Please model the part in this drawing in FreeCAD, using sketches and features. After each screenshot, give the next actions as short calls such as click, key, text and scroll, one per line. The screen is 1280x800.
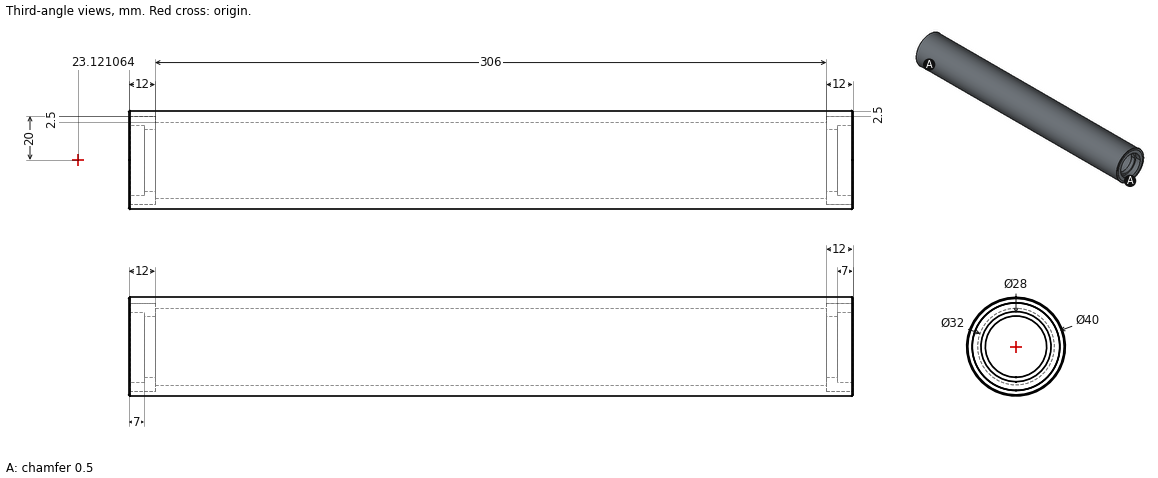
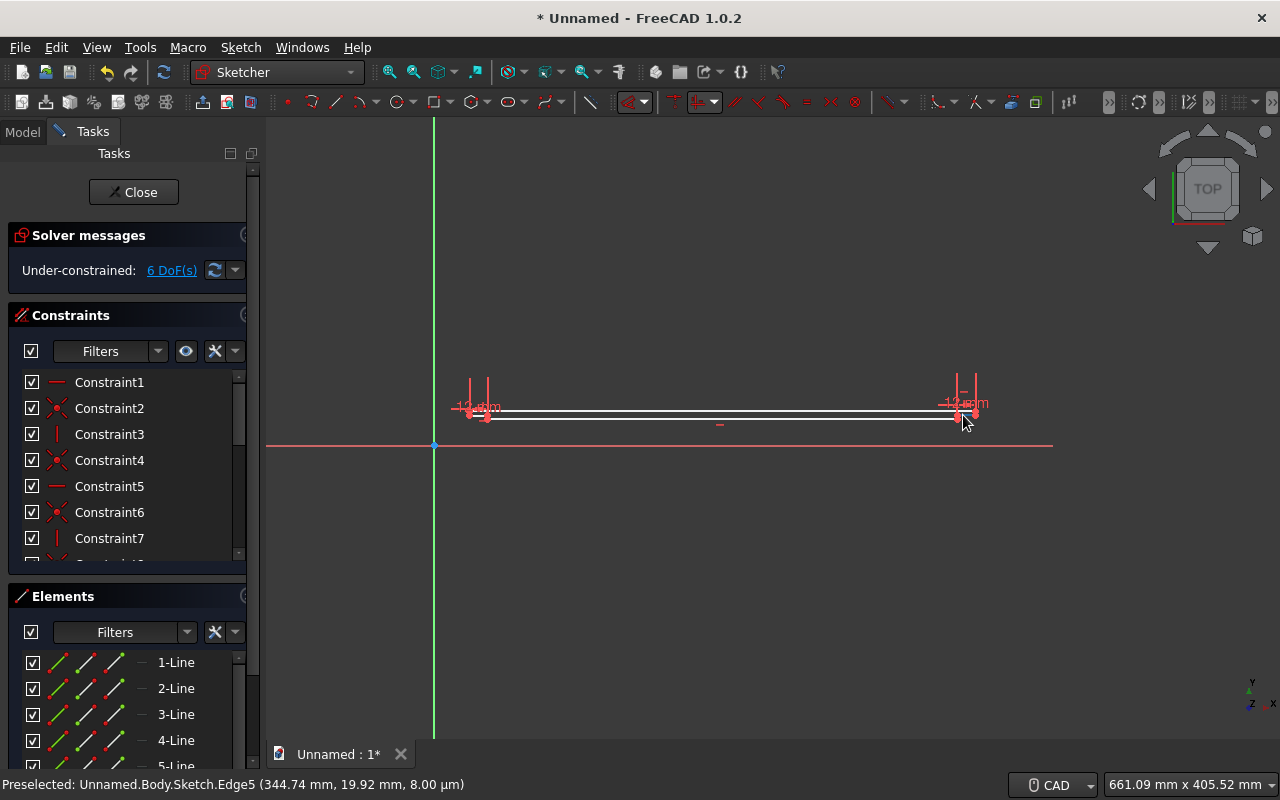
scroll(488, 418, up, 12)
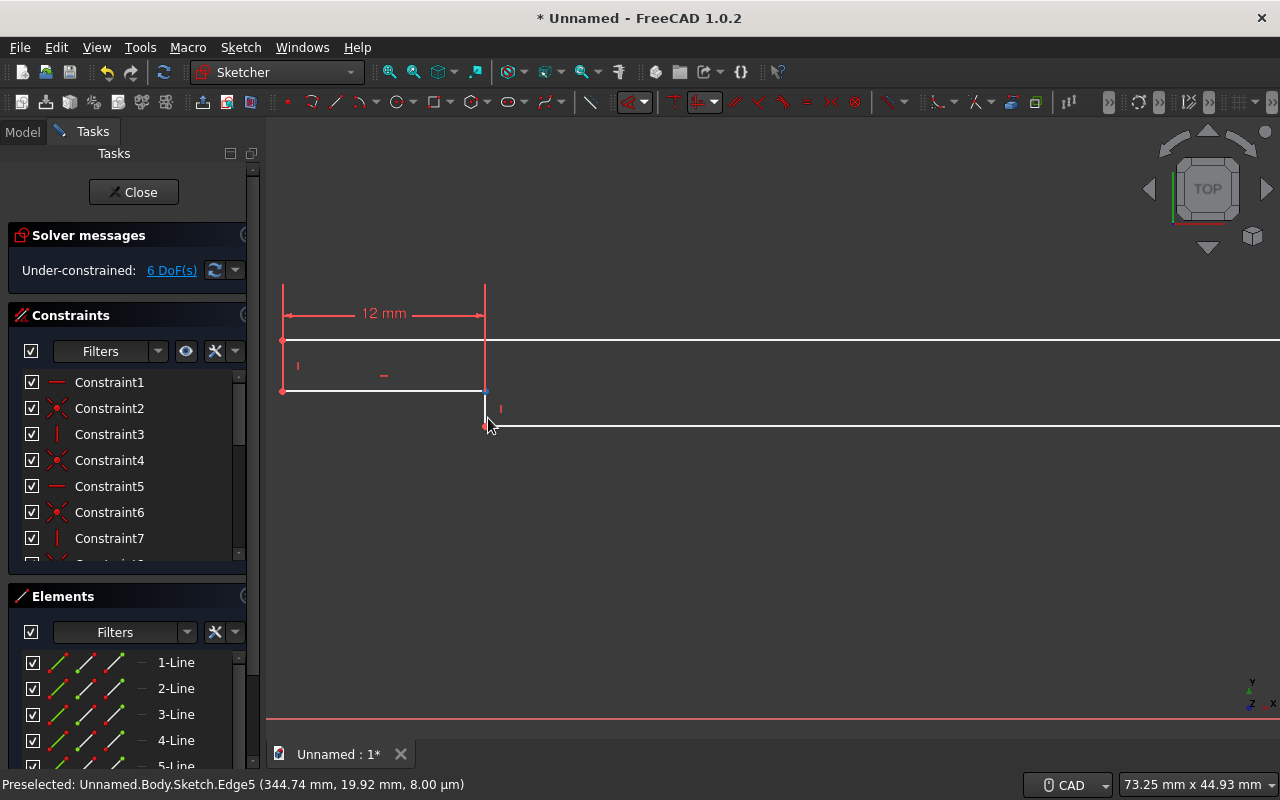
click(485, 409)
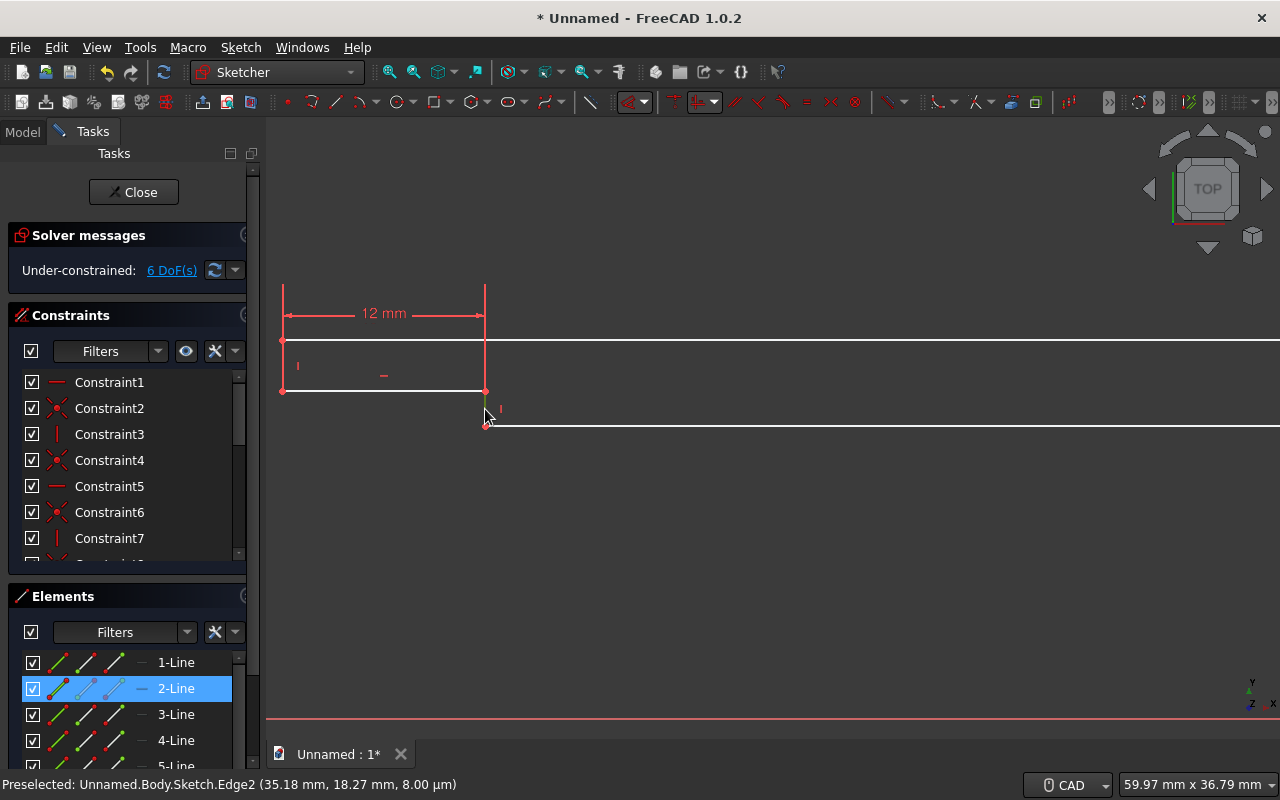
click(646, 102)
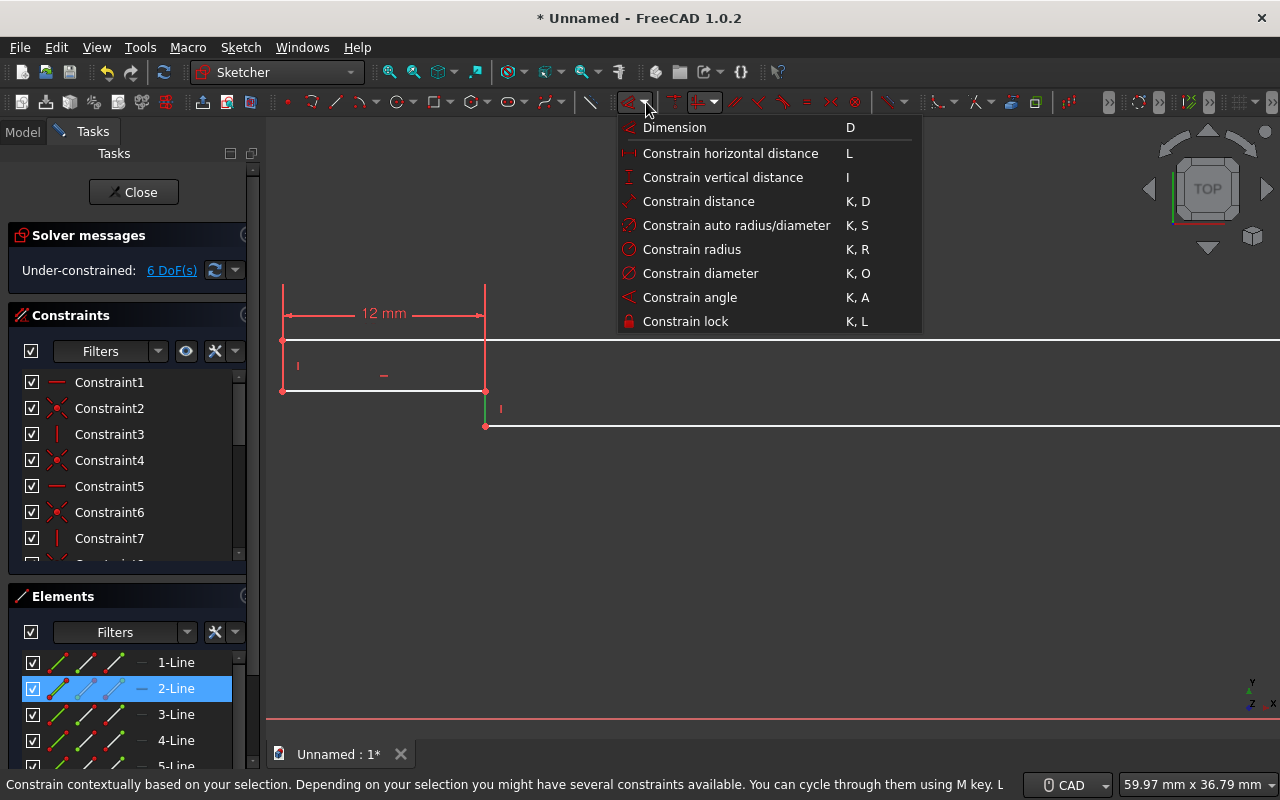
click(770, 177)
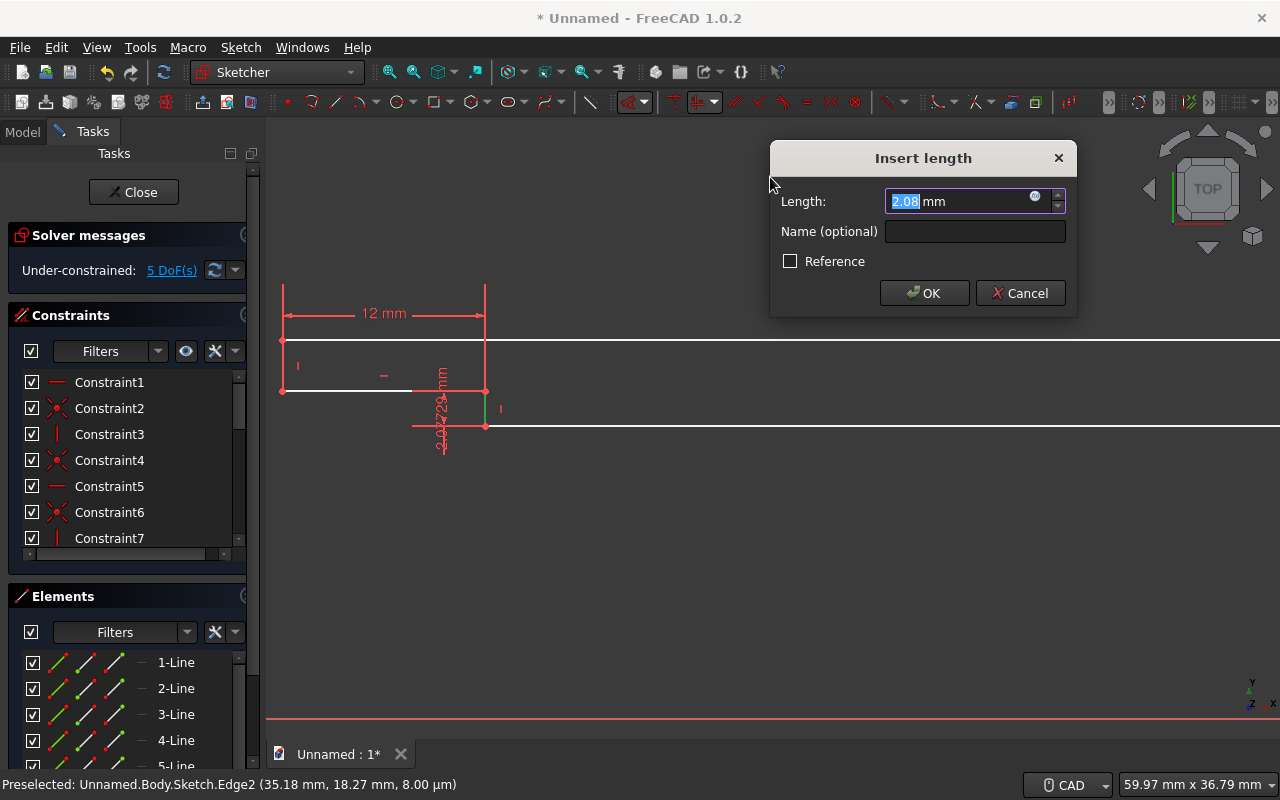
text(2.5)
key(Return)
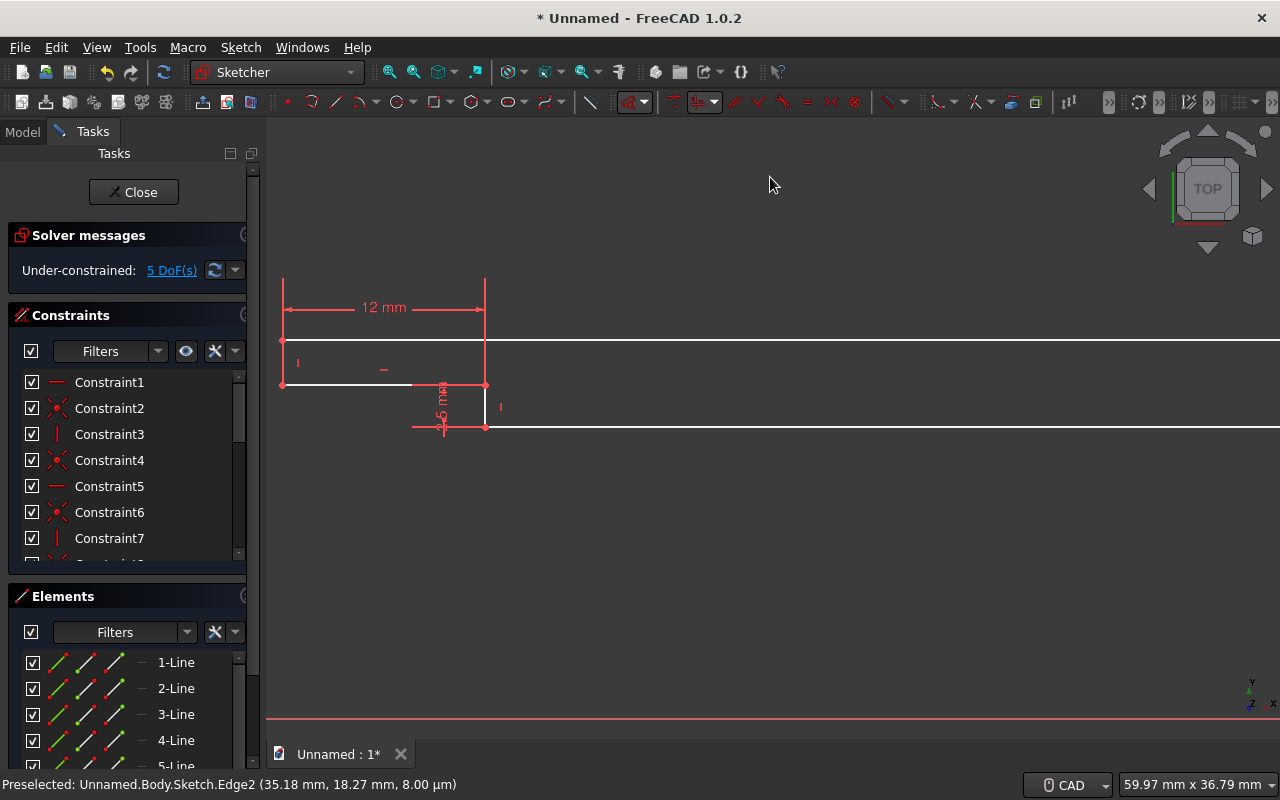
scroll(488, 418, down, 12)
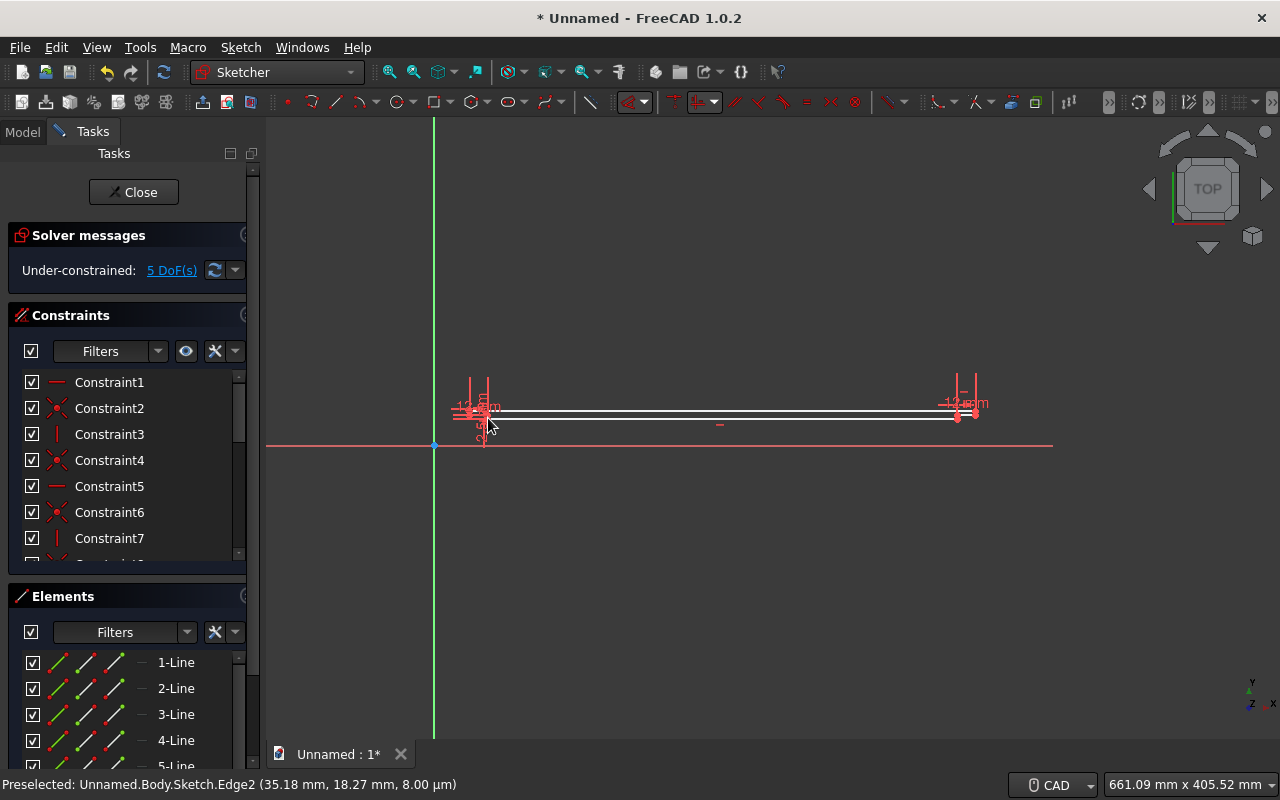
scroll(629, 419, up, 3)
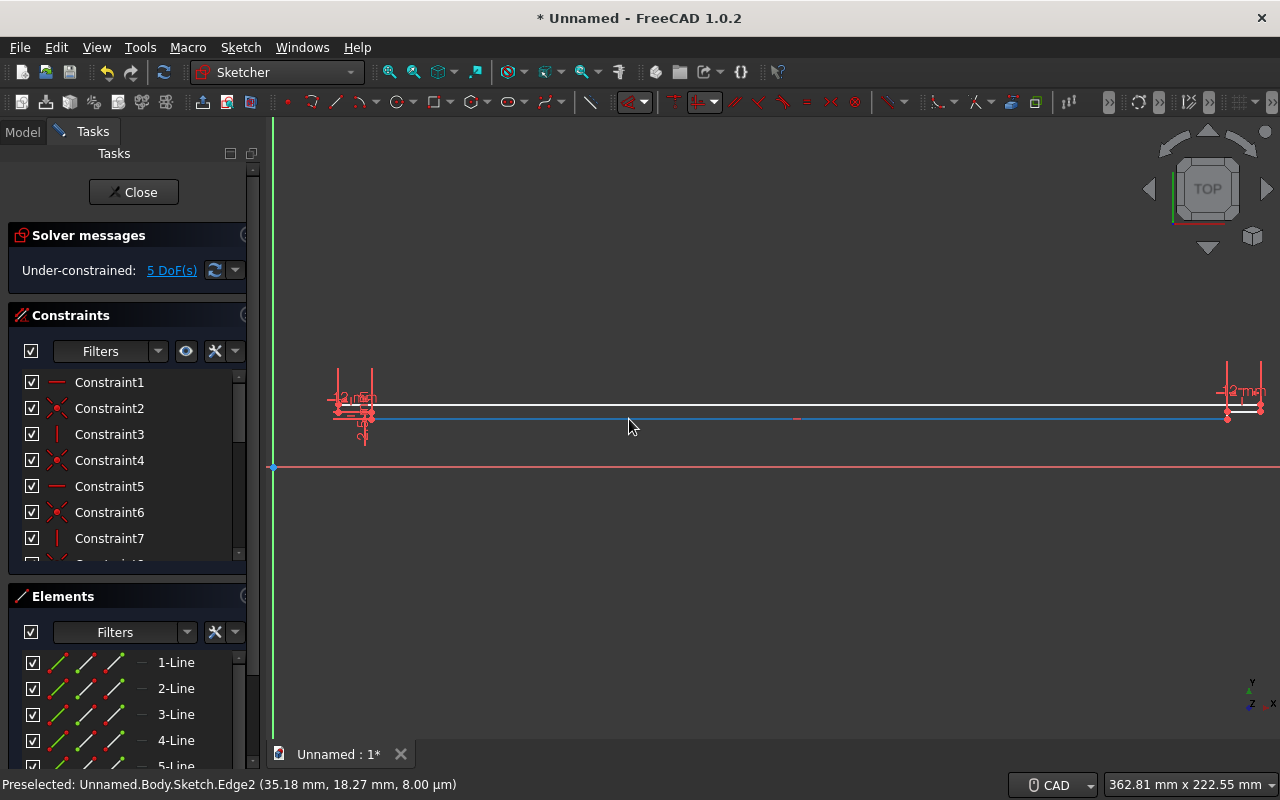
click(628, 419)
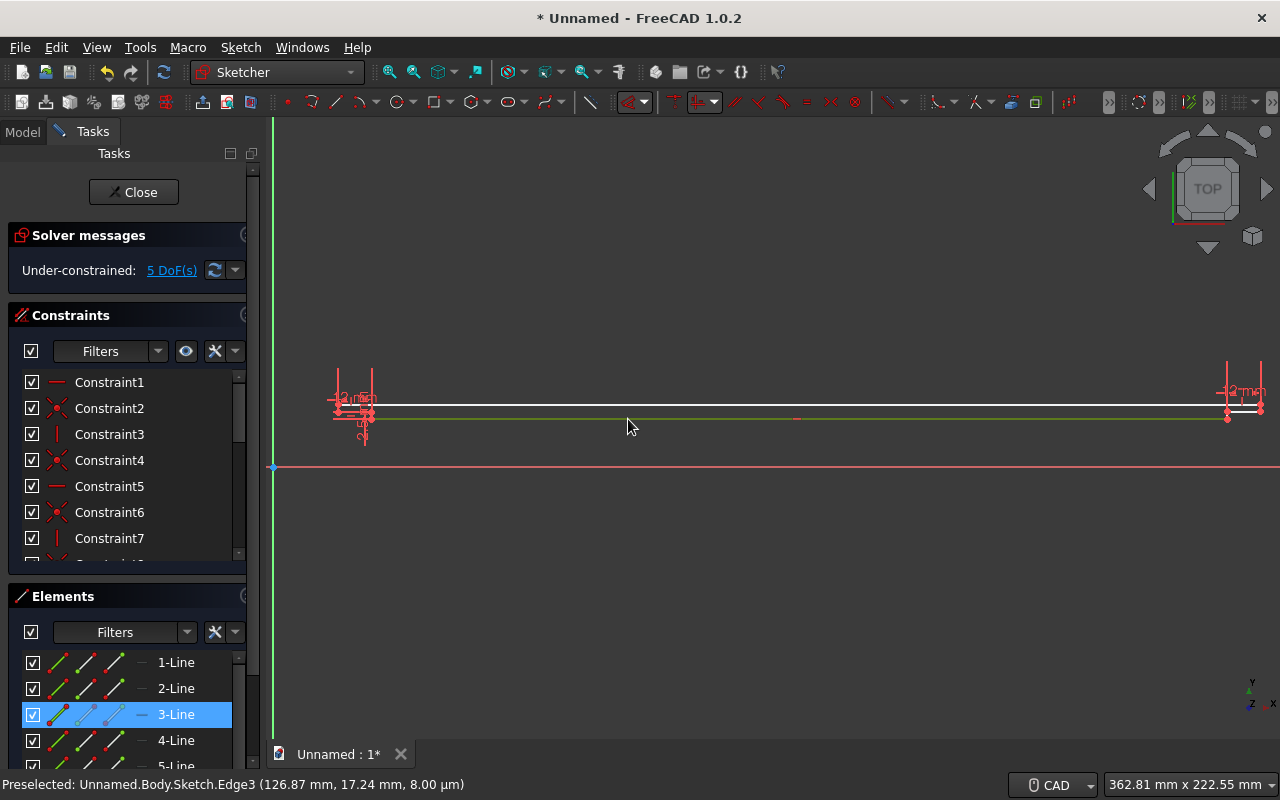
click(646, 102)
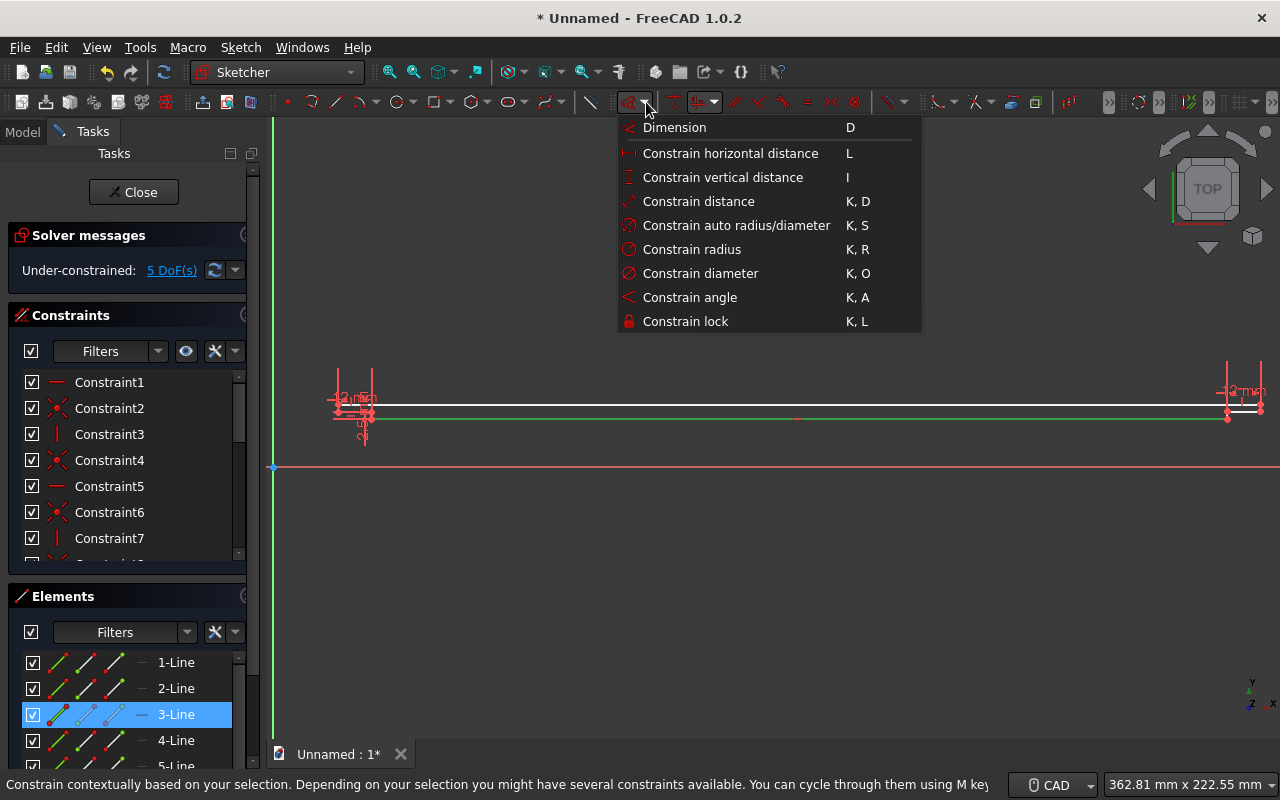
click(770, 153)